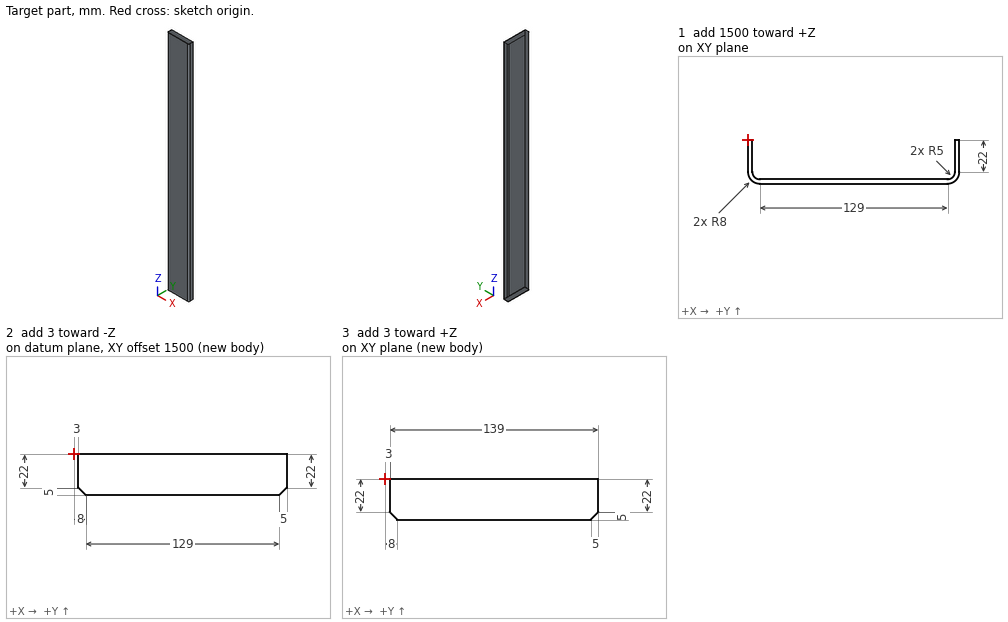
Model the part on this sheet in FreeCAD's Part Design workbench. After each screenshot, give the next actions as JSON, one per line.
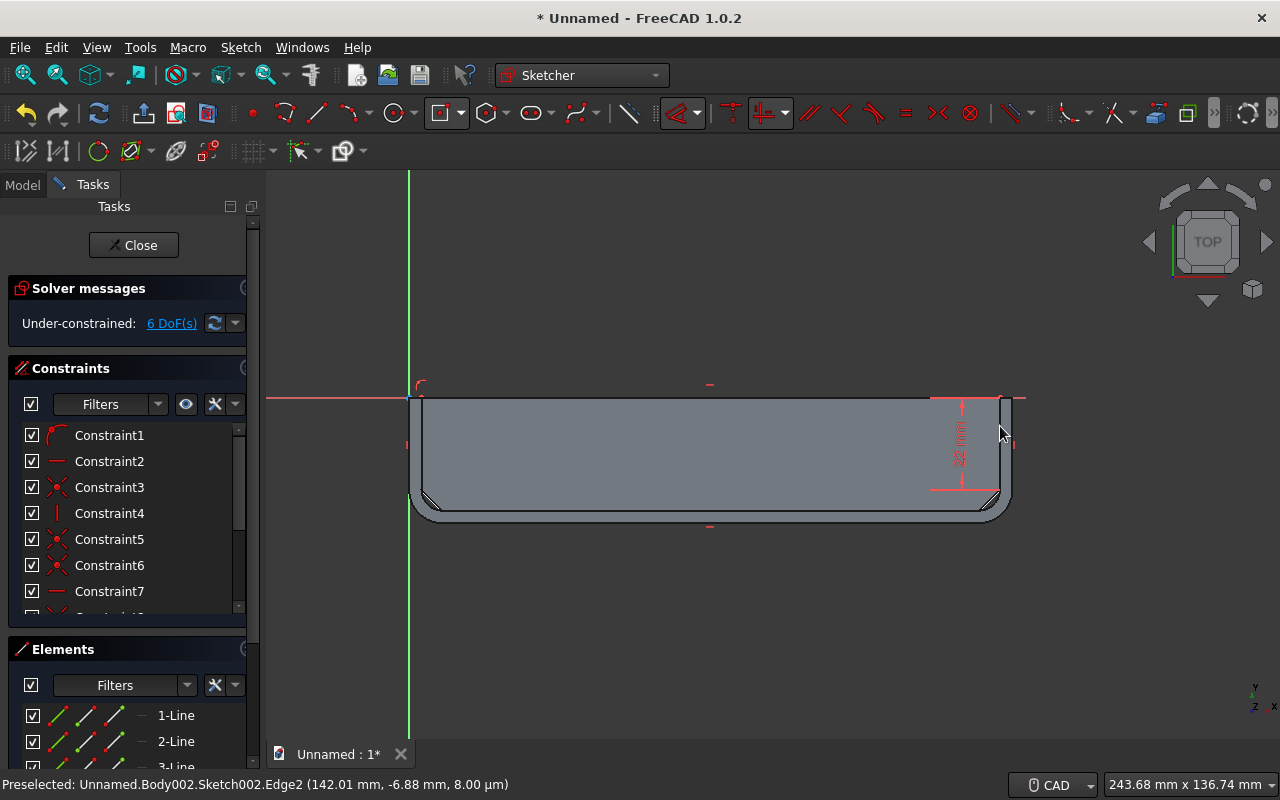
{"action": "left_click", "coordinate": [421, 463]}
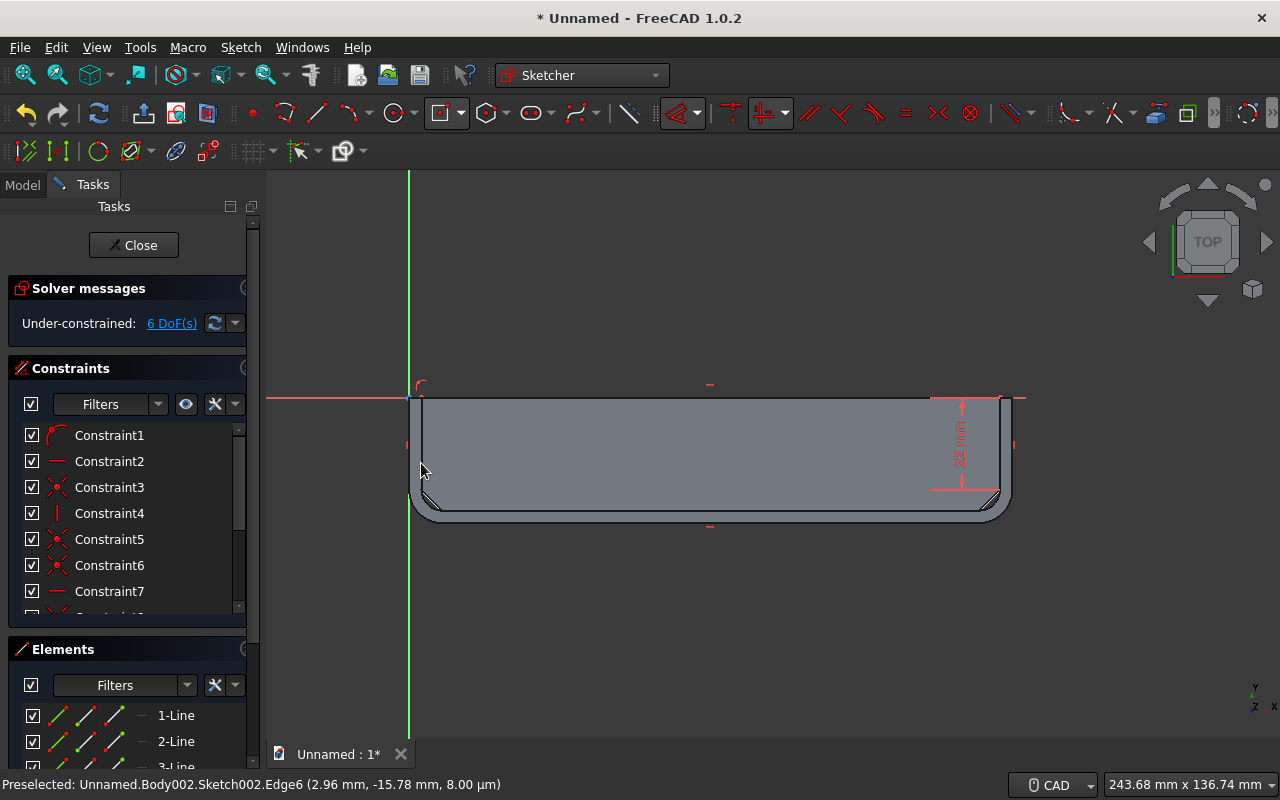
{"action": "key", "text": "i"}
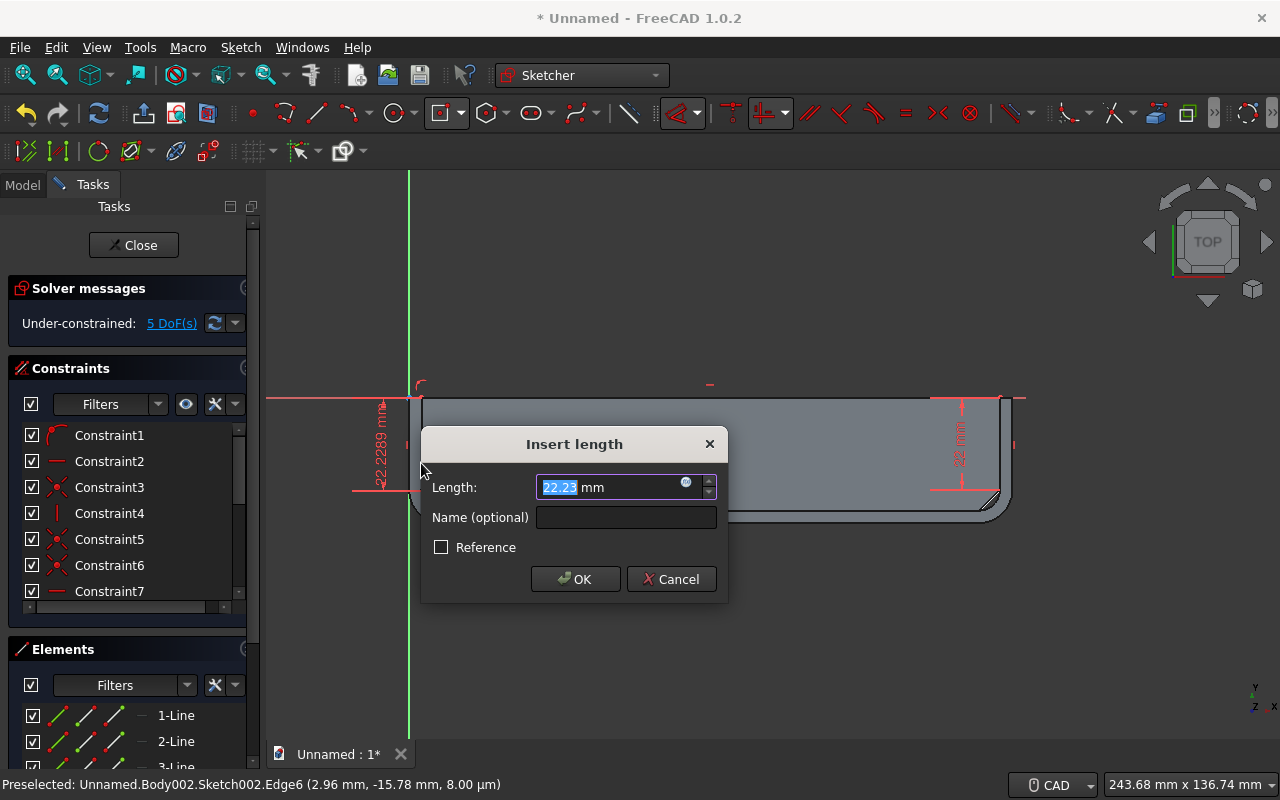
{"action": "type", "text": "22"}
{"action": "key", "text": "Return"}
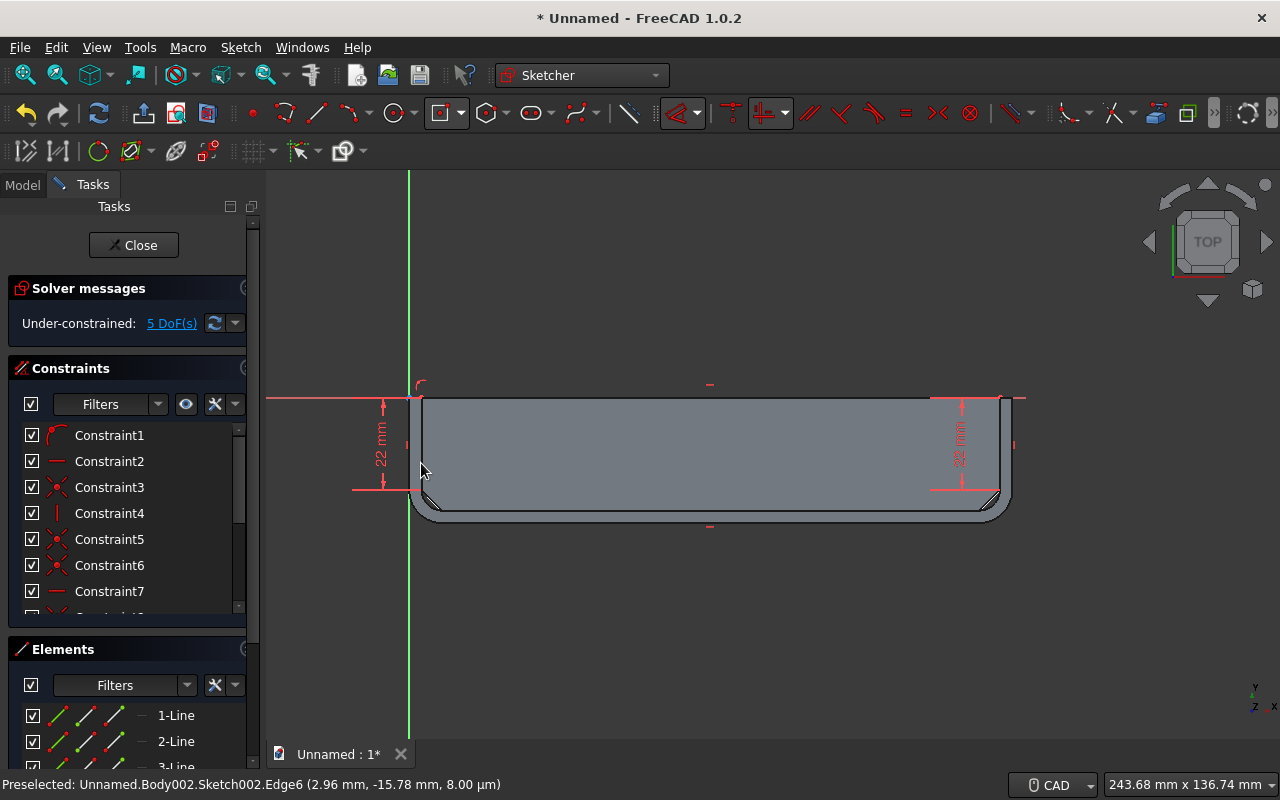
{"action": "scroll", "coordinate": [421, 398], "scroll_direction": "up", "scroll_amount": 6}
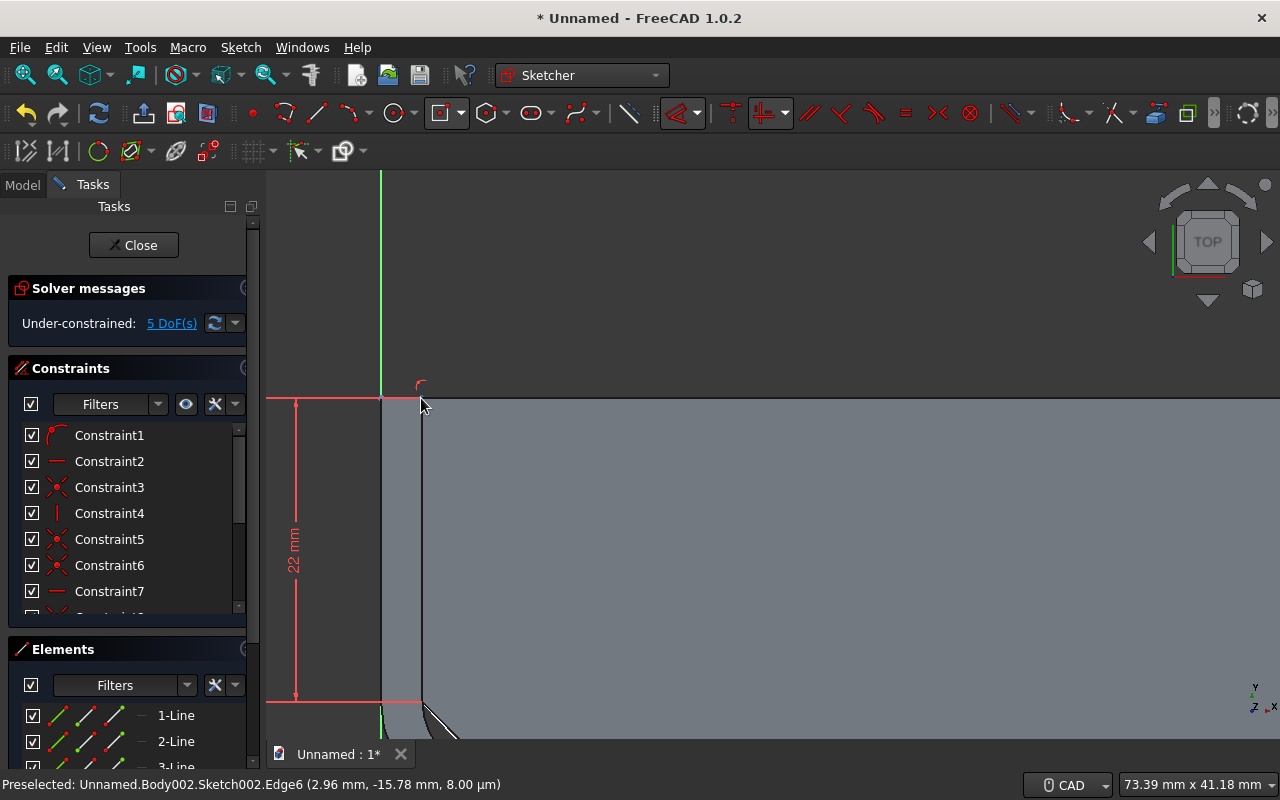
{"action": "left_click", "coordinate": [422, 398]}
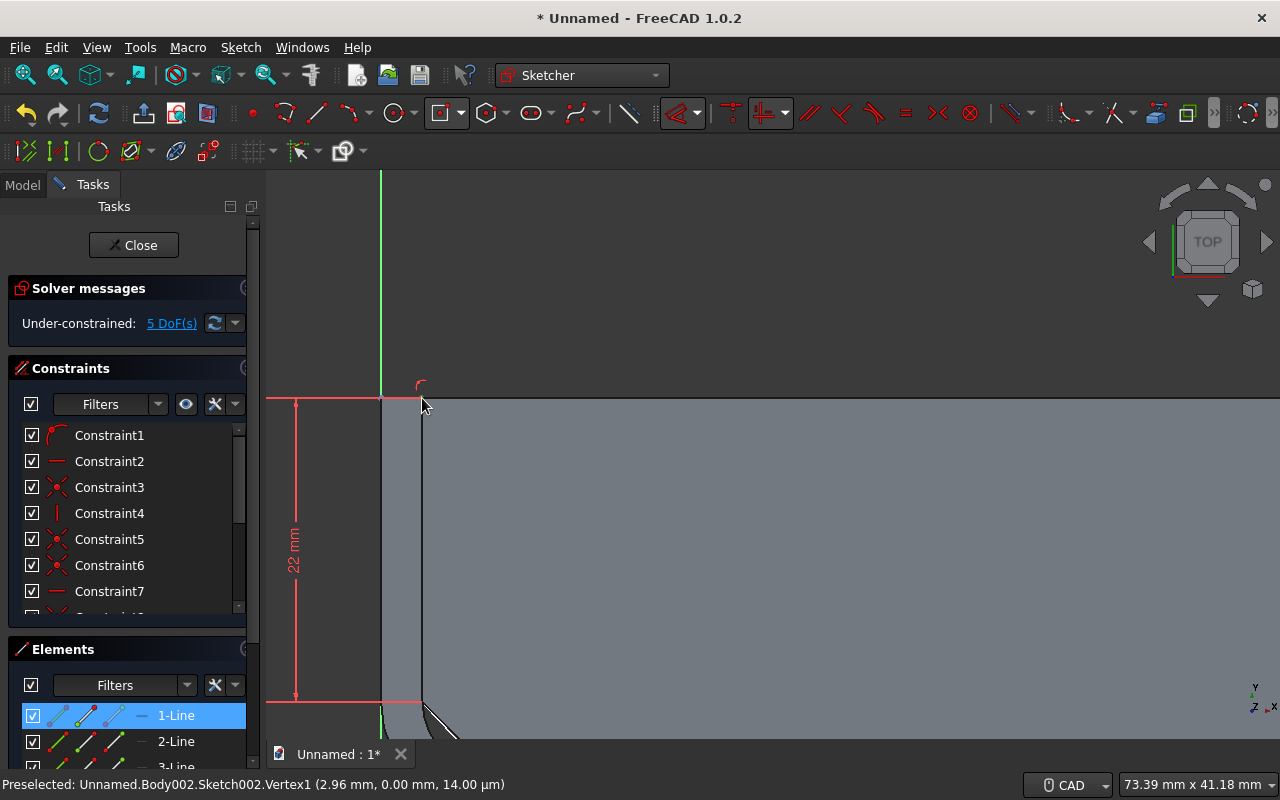
{"action": "key", "text": "l"}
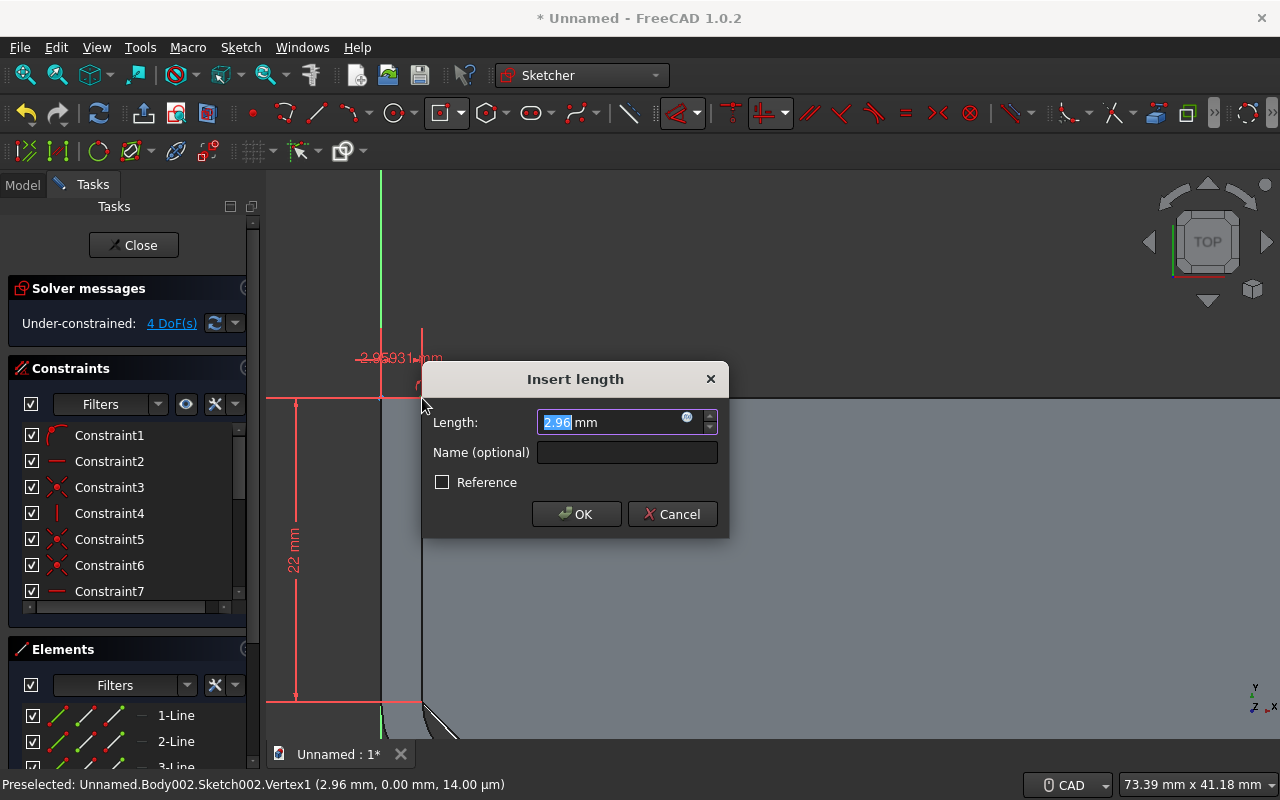
{"action": "type", "text": "3"}
{"action": "key", "text": "Return"}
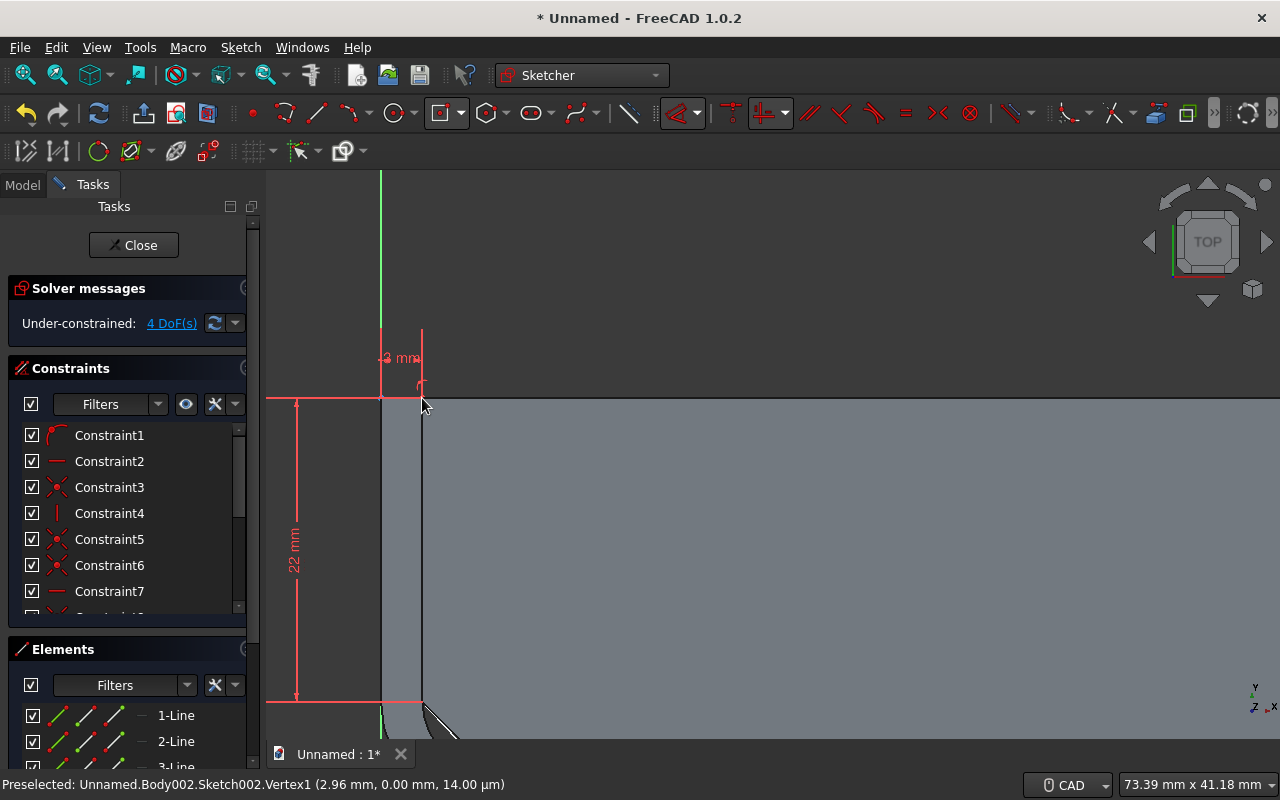
{"action": "scroll", "coordinate": [421, 398], "scroll_direction": "down", "scroll_amount": 6}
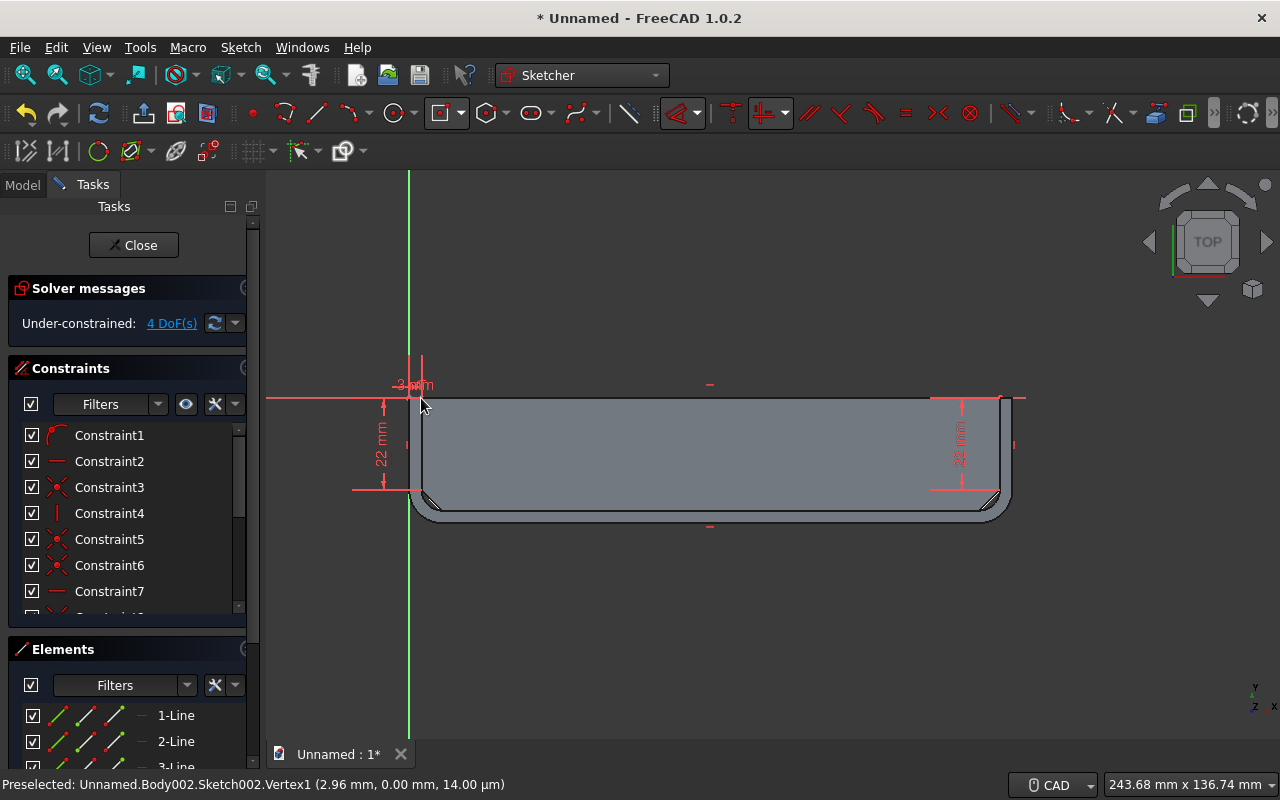
{"action": "left_click", "coordinate": [442, 512]}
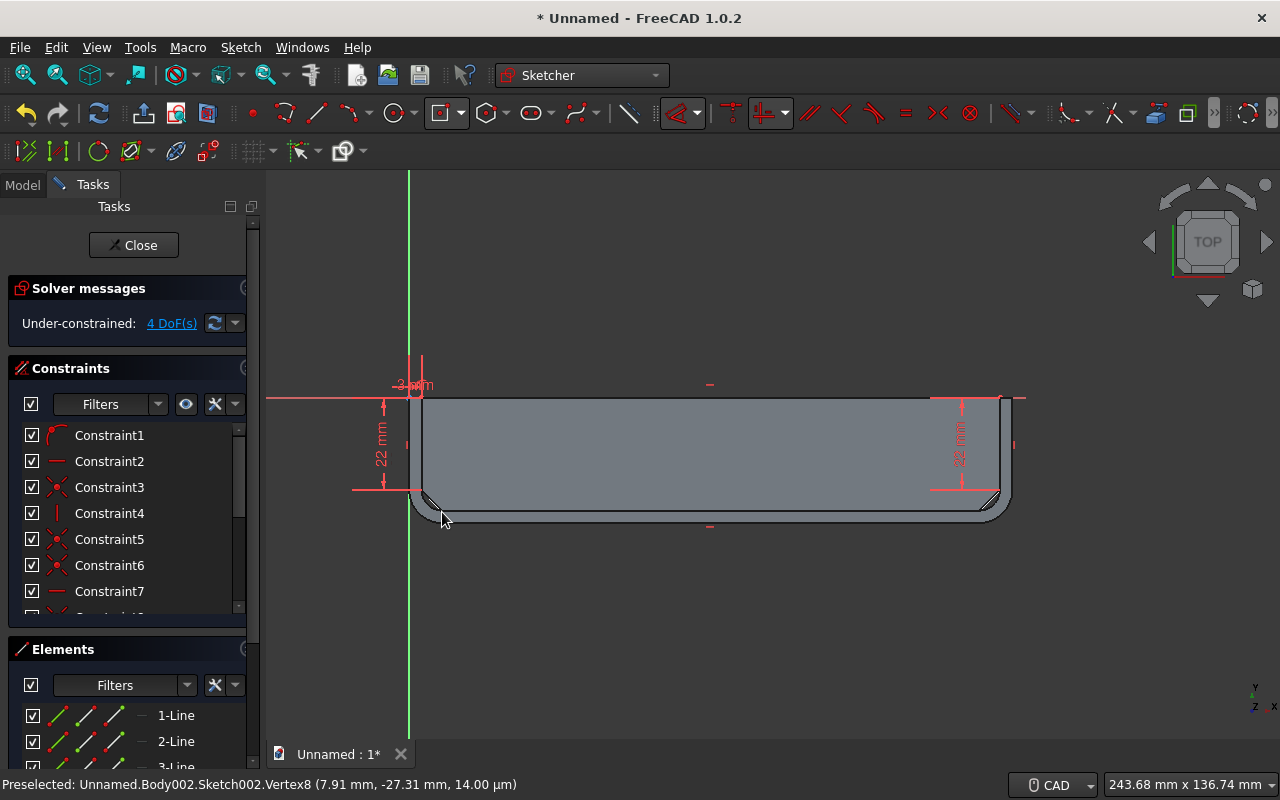
{"action": "left_click", "coordinate": [700, 114]}